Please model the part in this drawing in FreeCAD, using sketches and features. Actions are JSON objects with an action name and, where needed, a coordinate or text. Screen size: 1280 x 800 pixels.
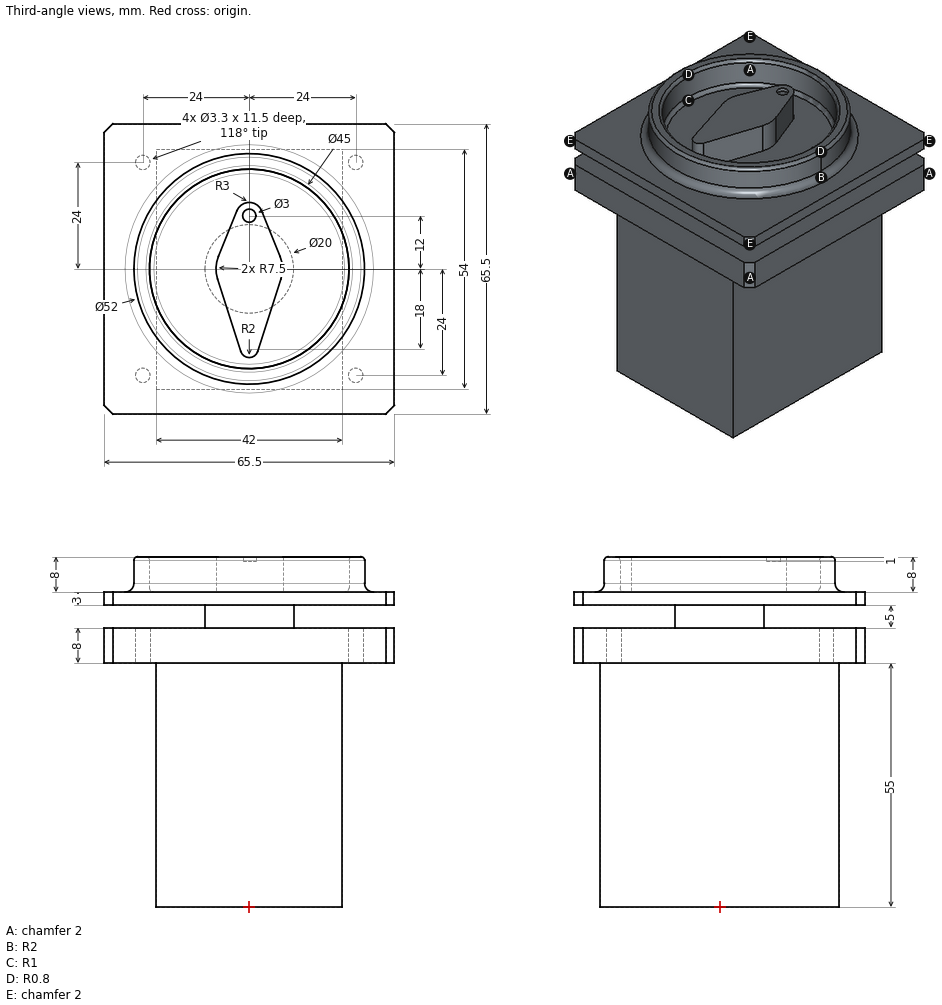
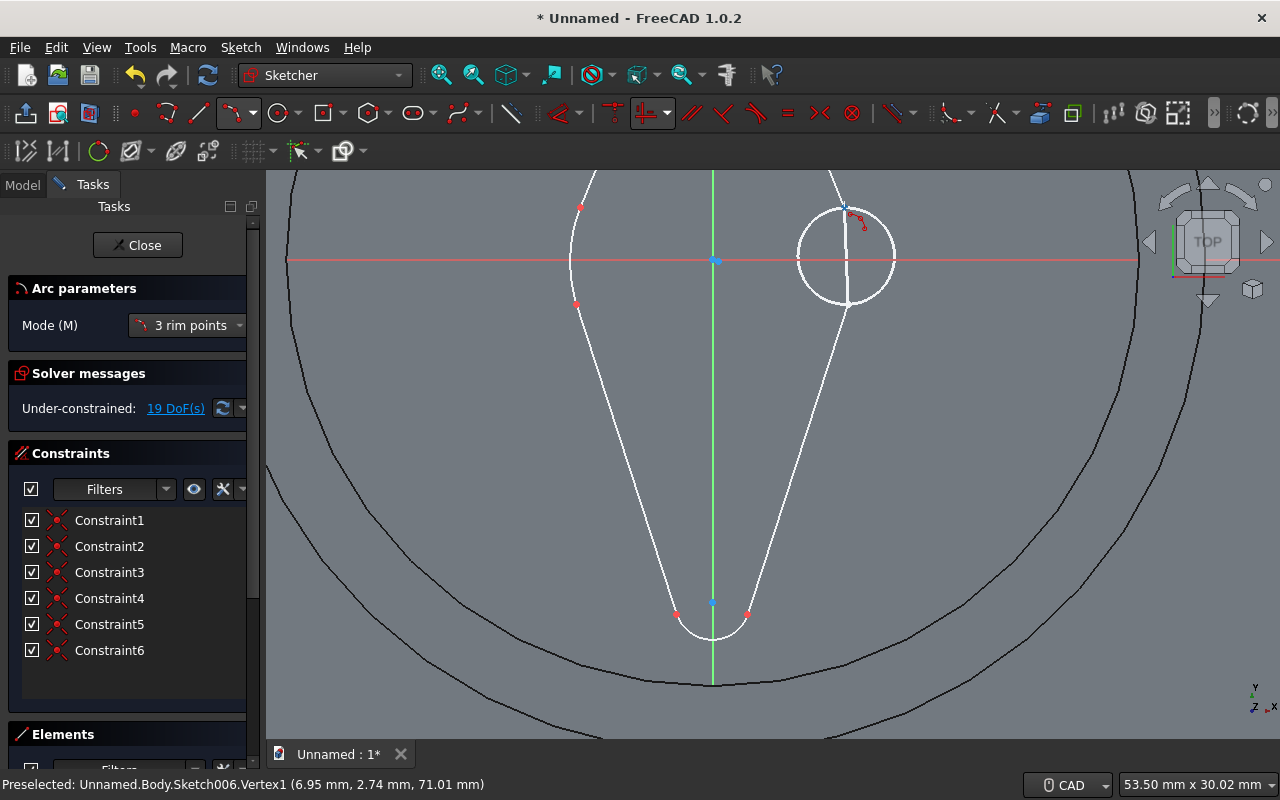
{"action": "scroll", "coordinate": [854, 245], "scroll_direction": "up", "scroll_amount": 4}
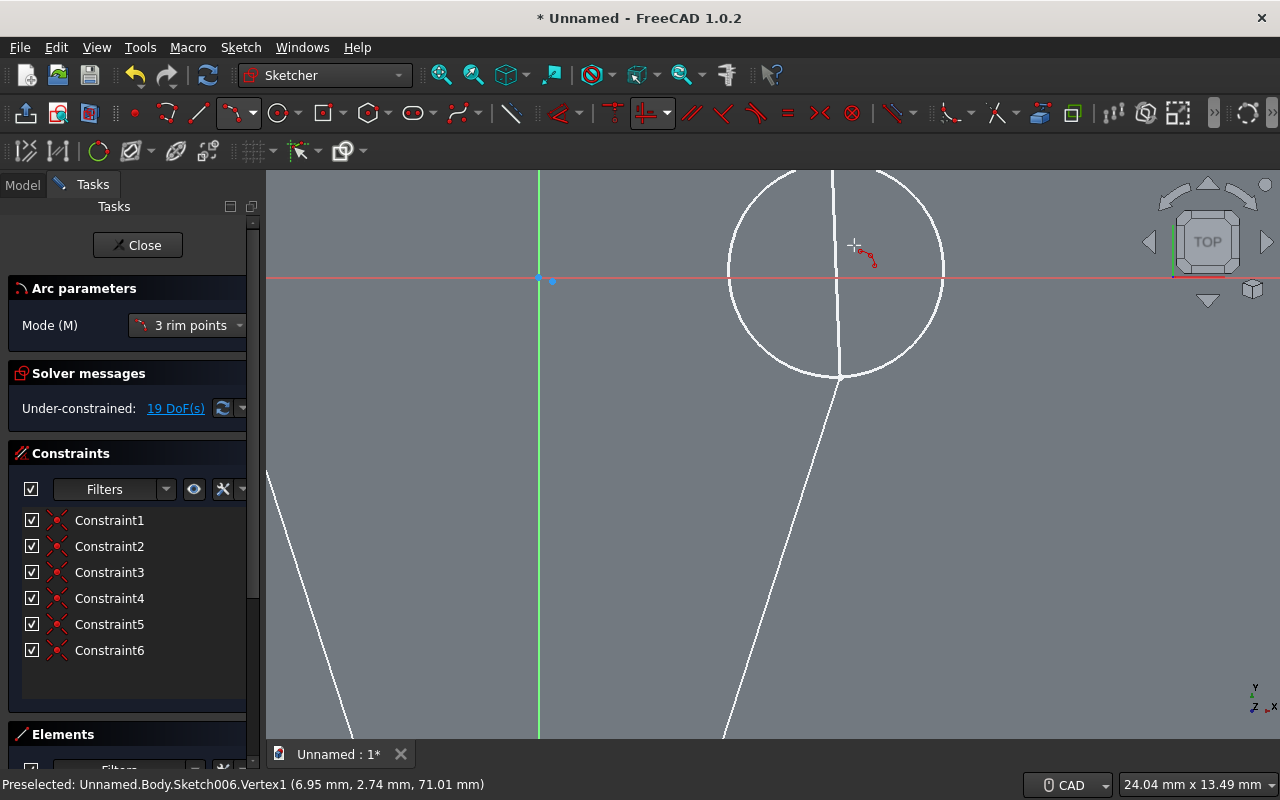
{"action": "left_click", "coordinate": [853, 244]}
{"action": "key", "text": "Escape"}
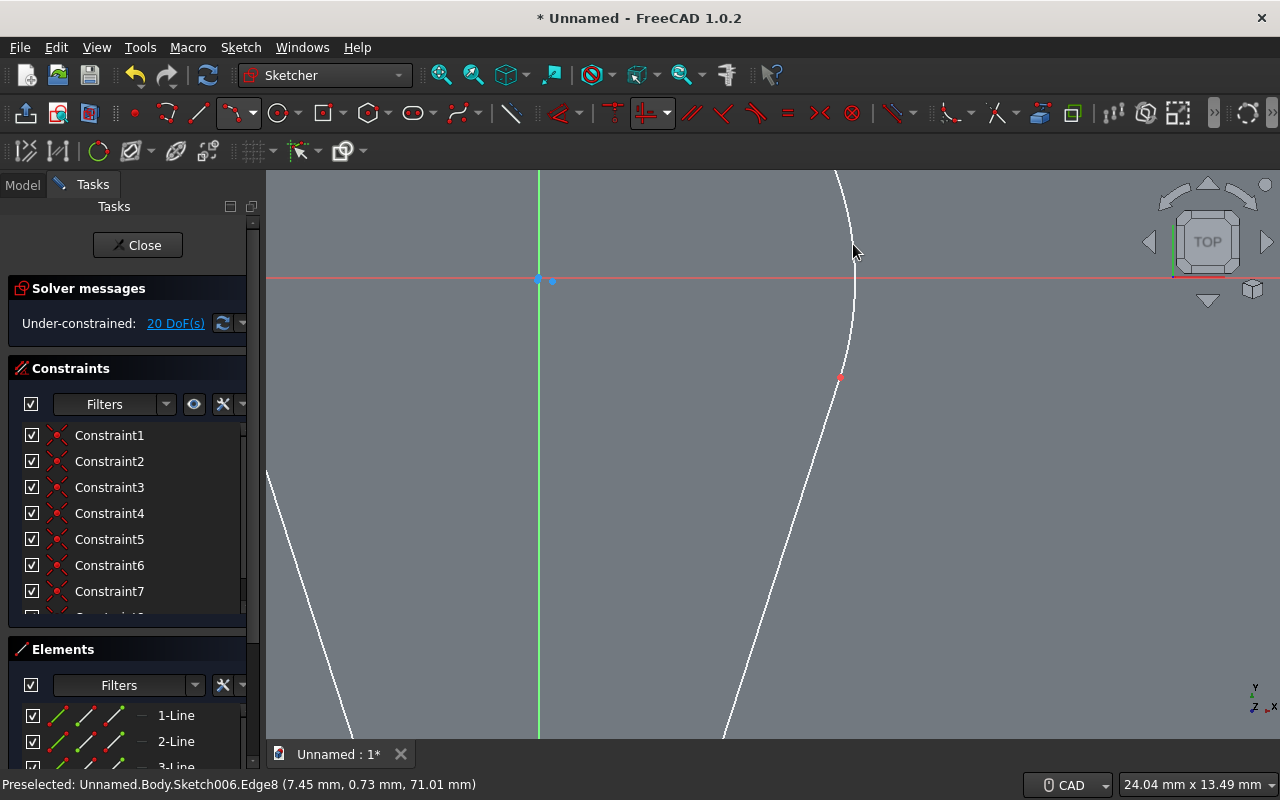
{"action": "scroll", "coordinate": [759, 478], "scroll_direction": "down", "scroll_amount": 7}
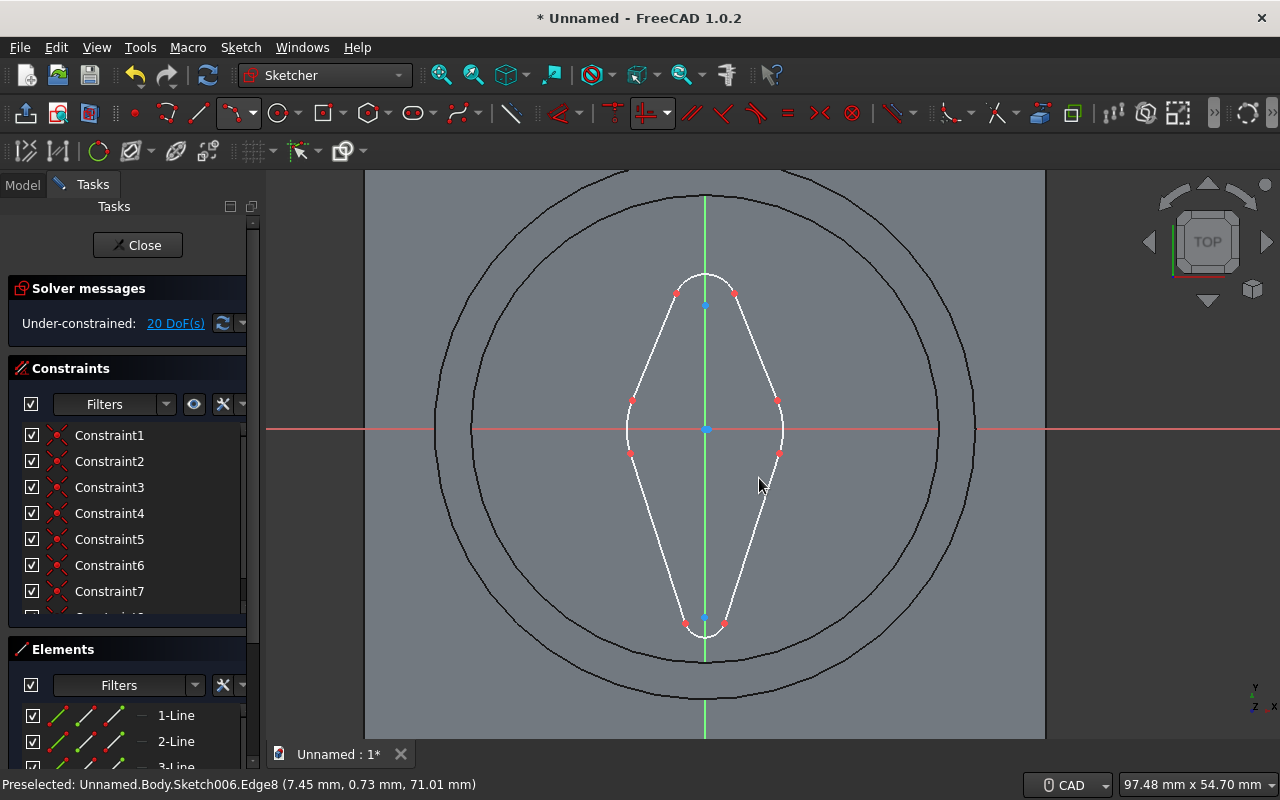
{"action": "left_click", "coordinate": [764, 368]}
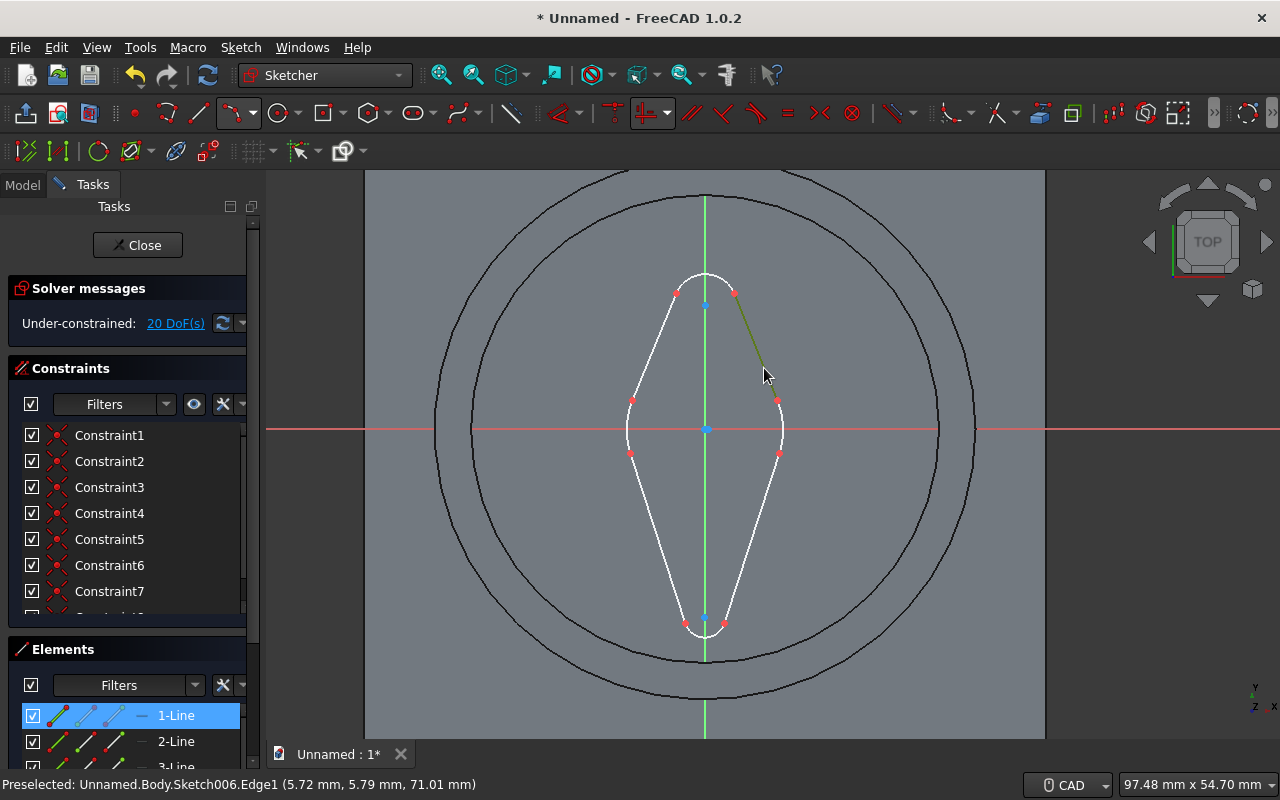
{"action": "left_click", "coordinate": [720, 278]}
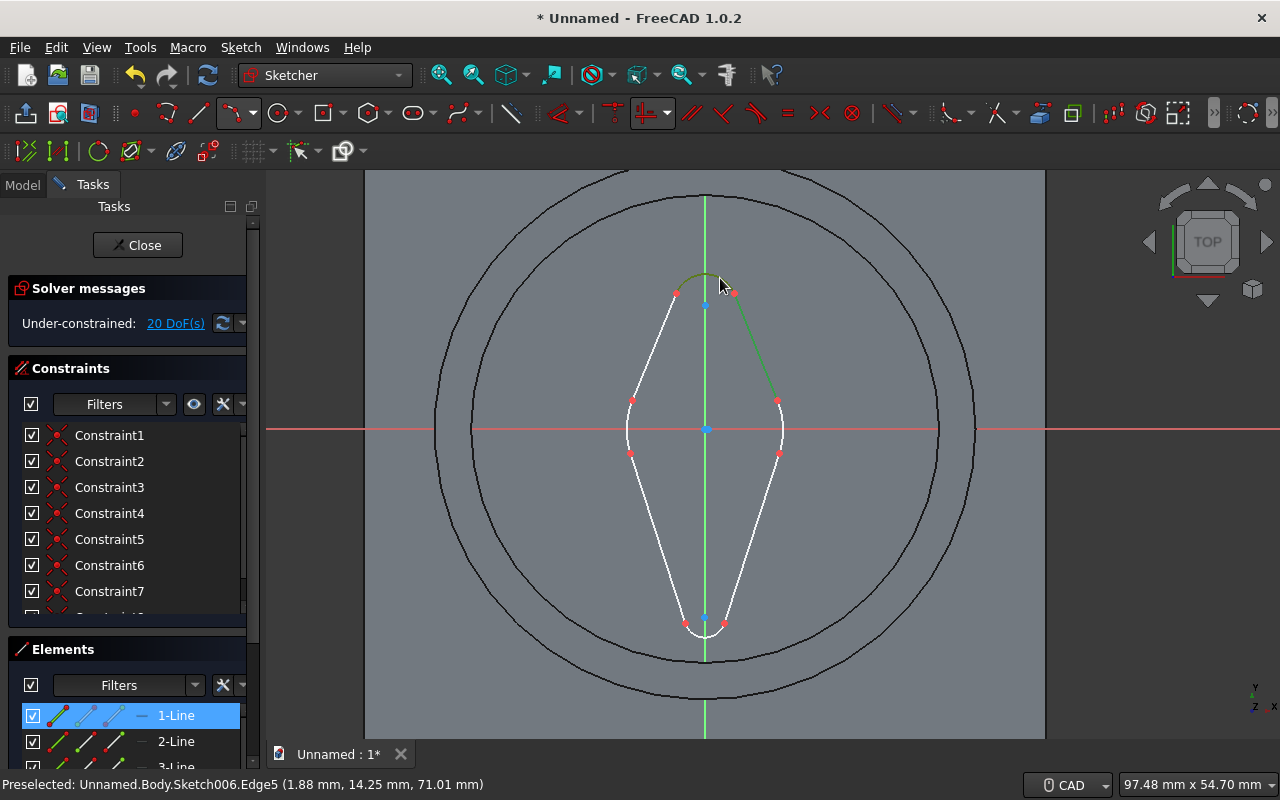
{"action": "left_click", "coordinate": [756, 114]}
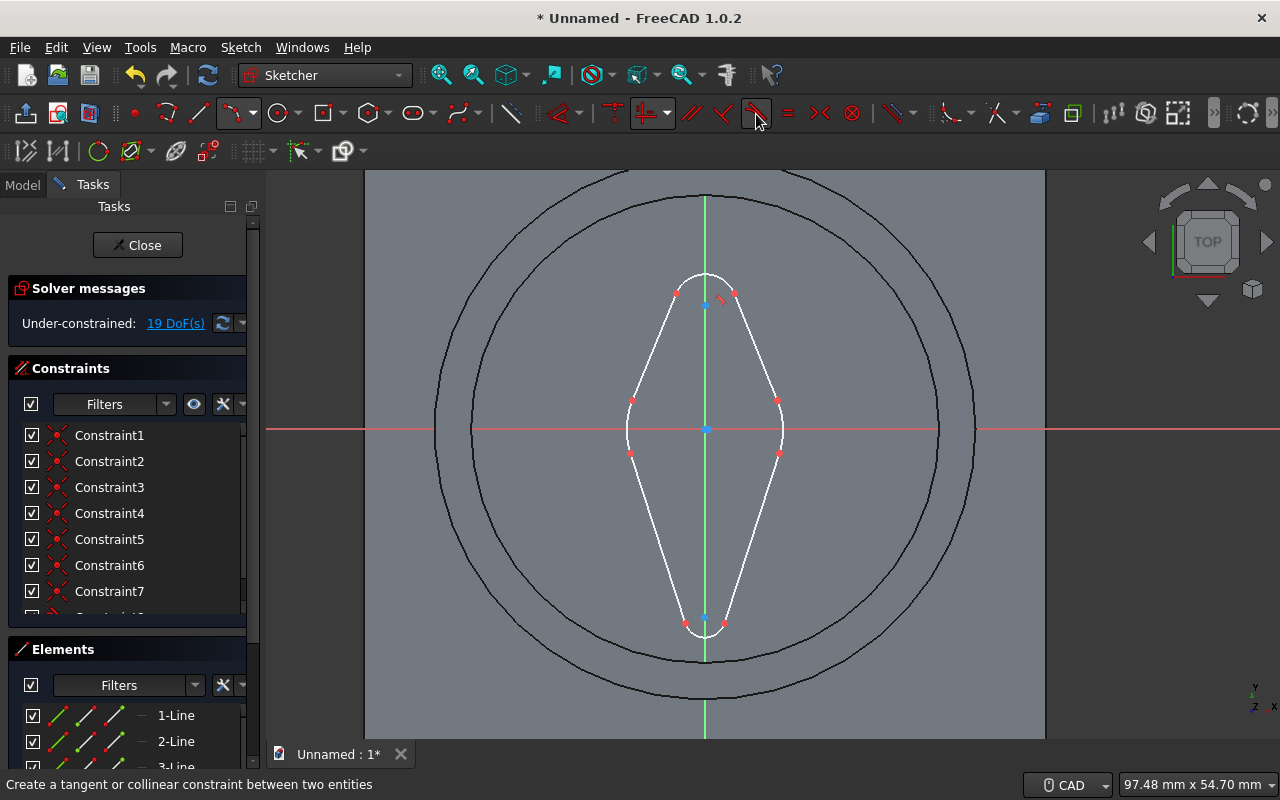
{"action": "left_click", "coordinate": [764, 369]}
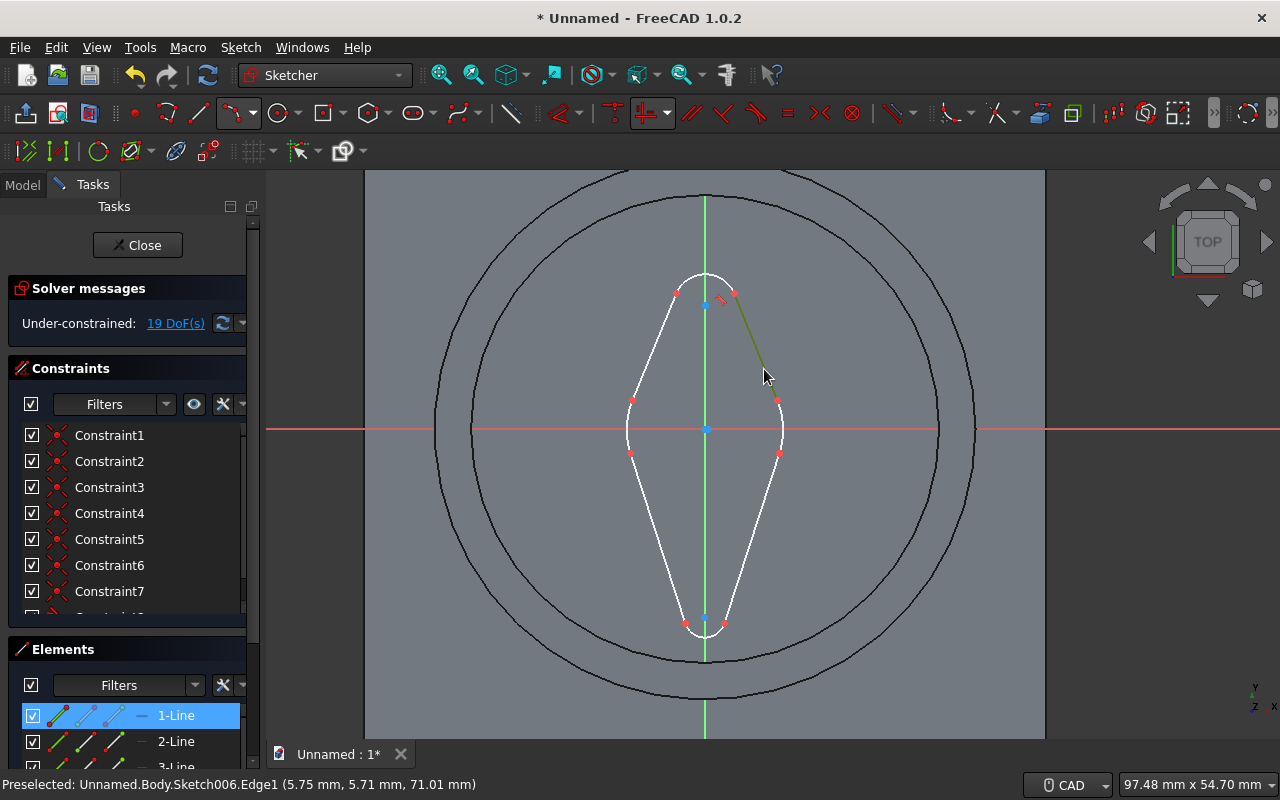
{"action": "left_click", "coordinate": [782, 416]}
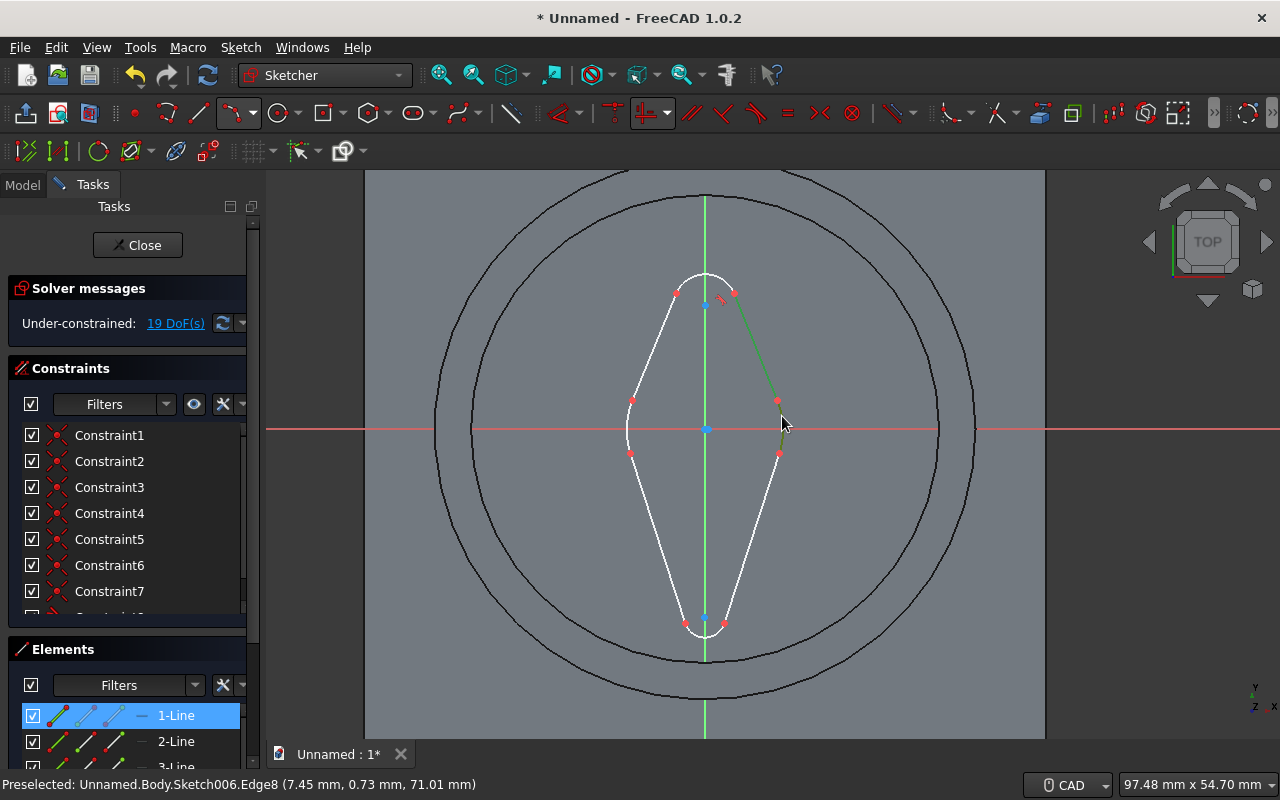
{"action": "left_click", "coordinate": [756, 114]}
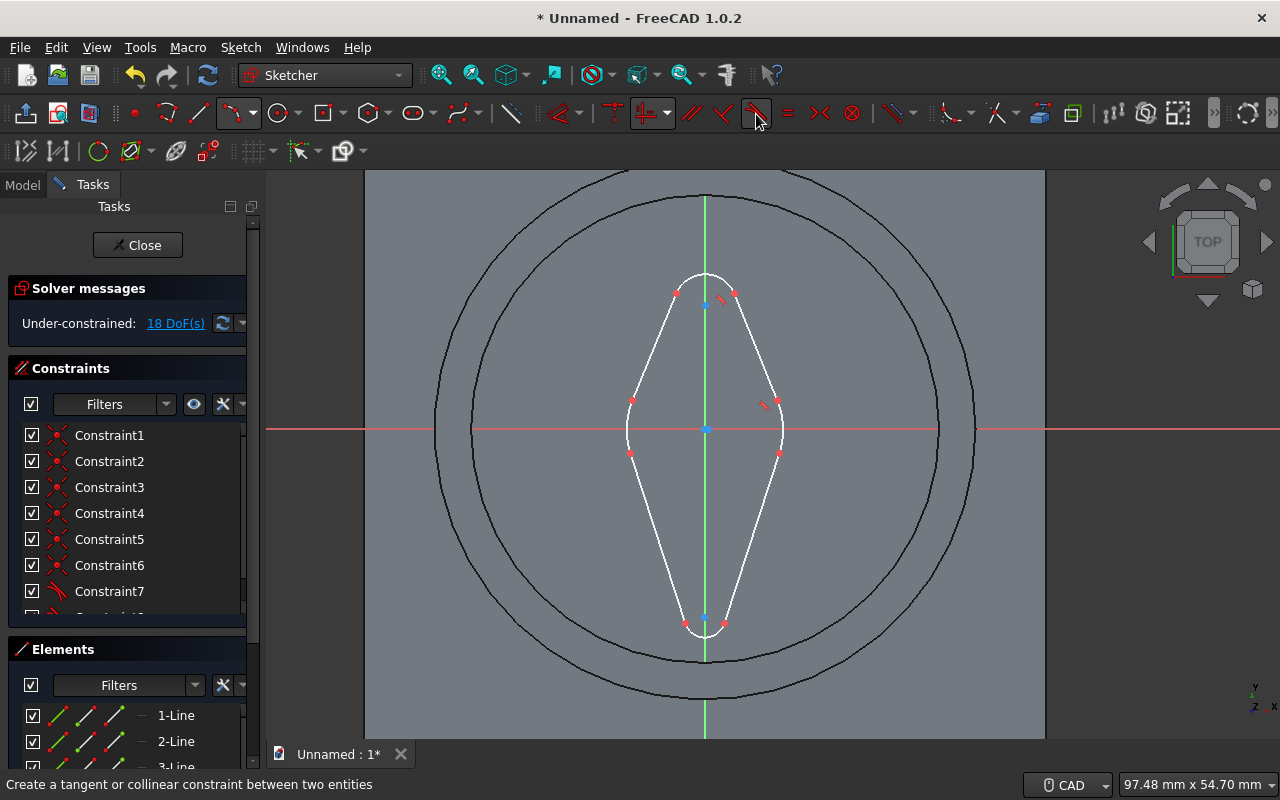
{"action": "left_click", "coordinate": [663, 326]}